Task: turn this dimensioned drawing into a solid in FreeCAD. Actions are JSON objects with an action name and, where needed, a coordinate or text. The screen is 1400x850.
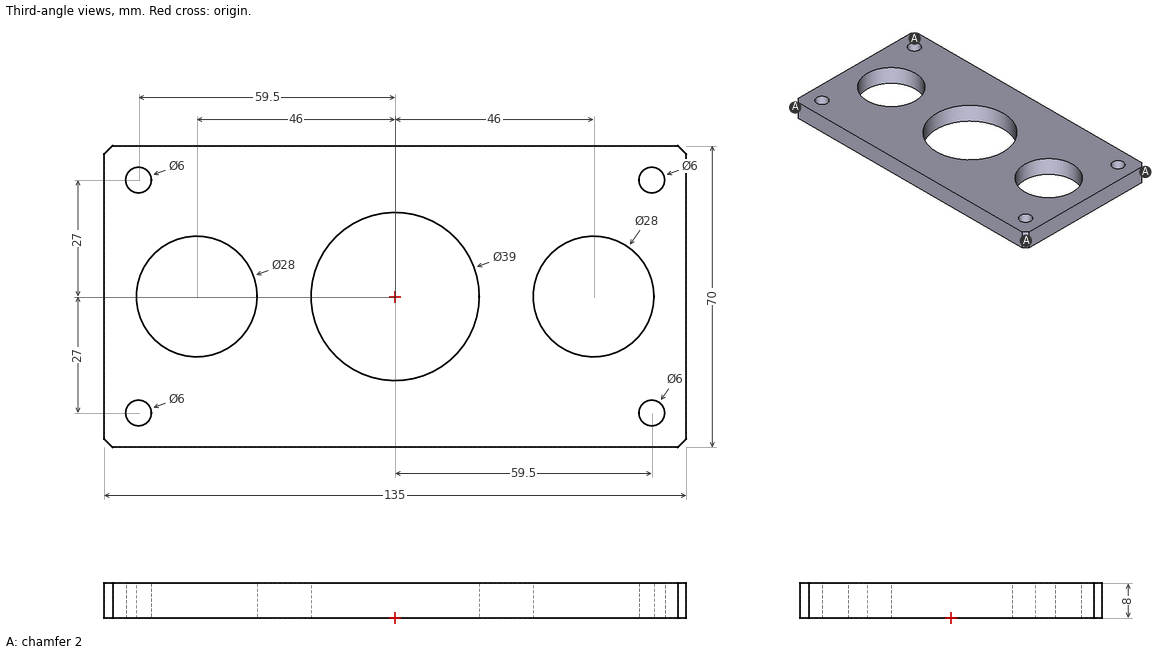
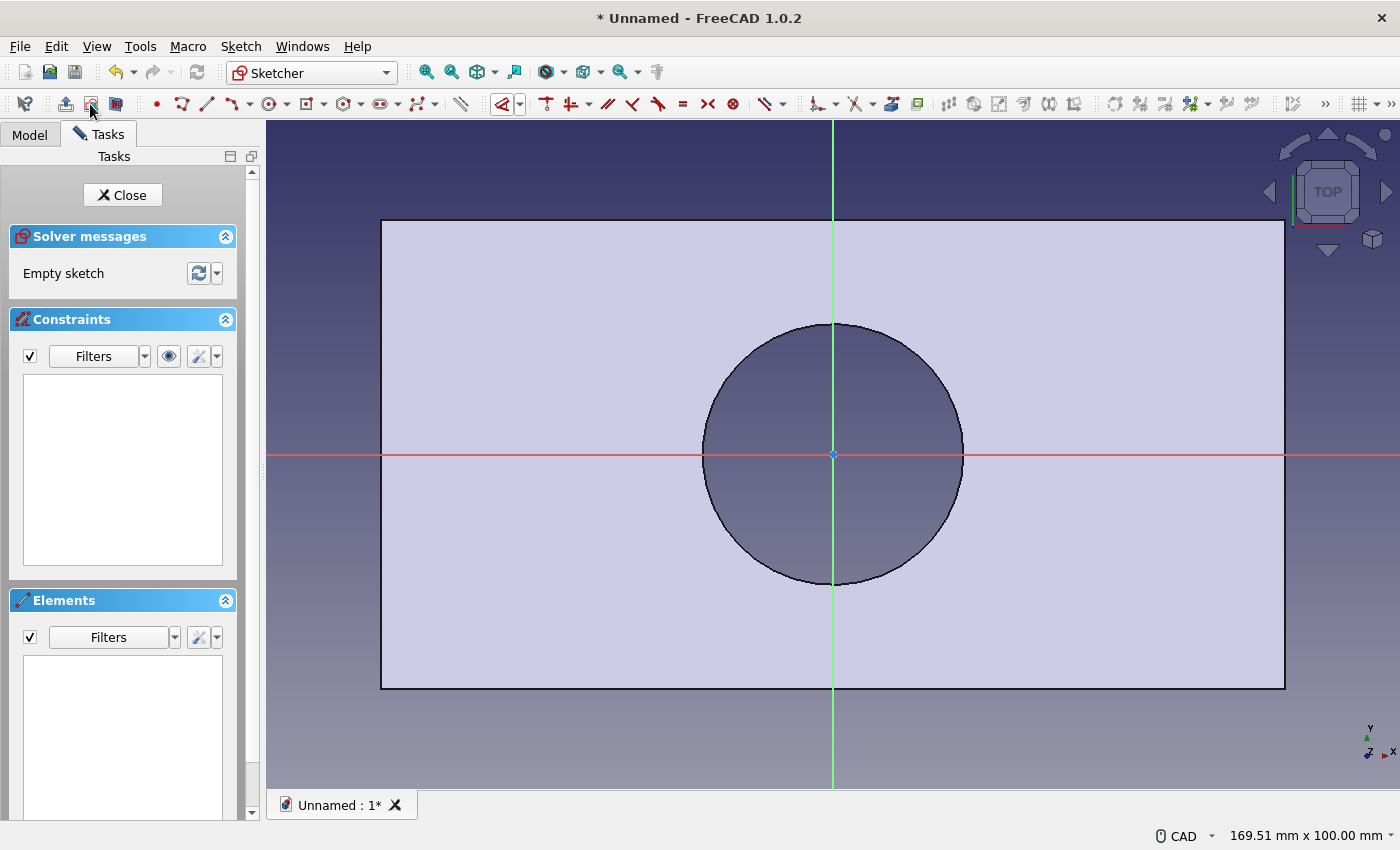
{"action": "scroll", "coordinate": [764, 454], "scroll_direction": "down", "scroll_amount": 5}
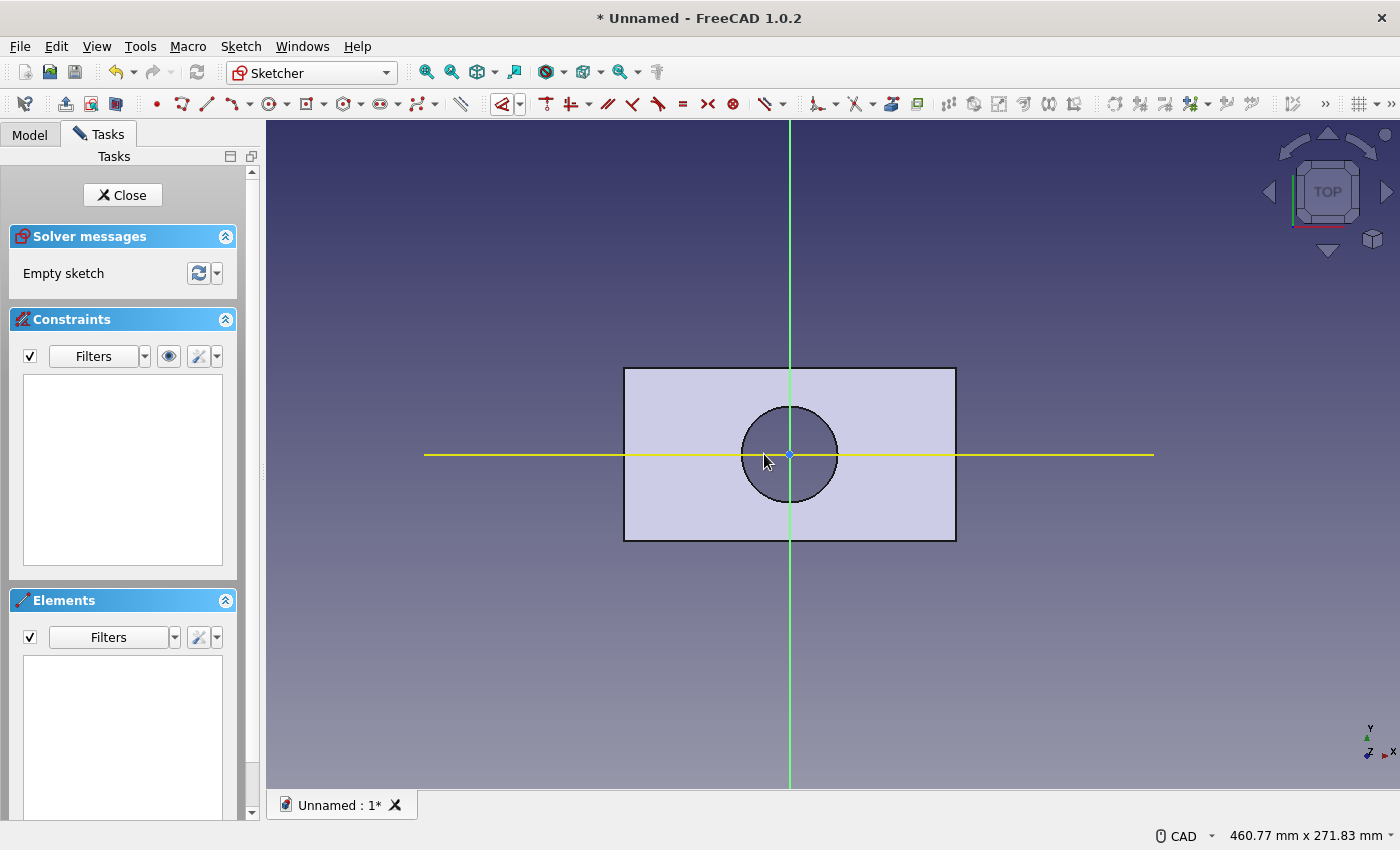
{"action": "scroll", "coordinate": [889, 454], "scroll_direction": "up", "scroll_amount": 8}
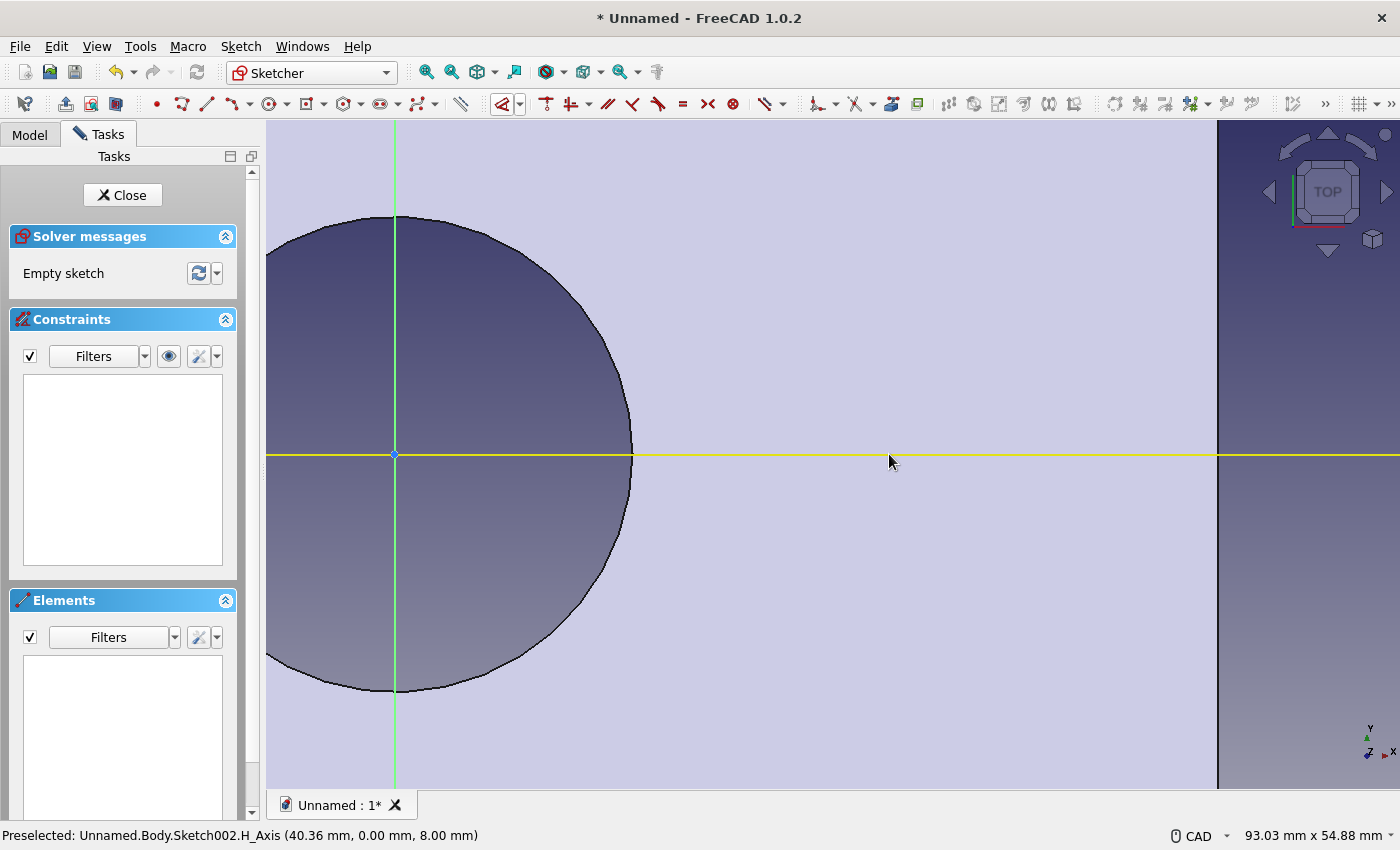
{"action": "left_click", "coordinate": [268, 104]}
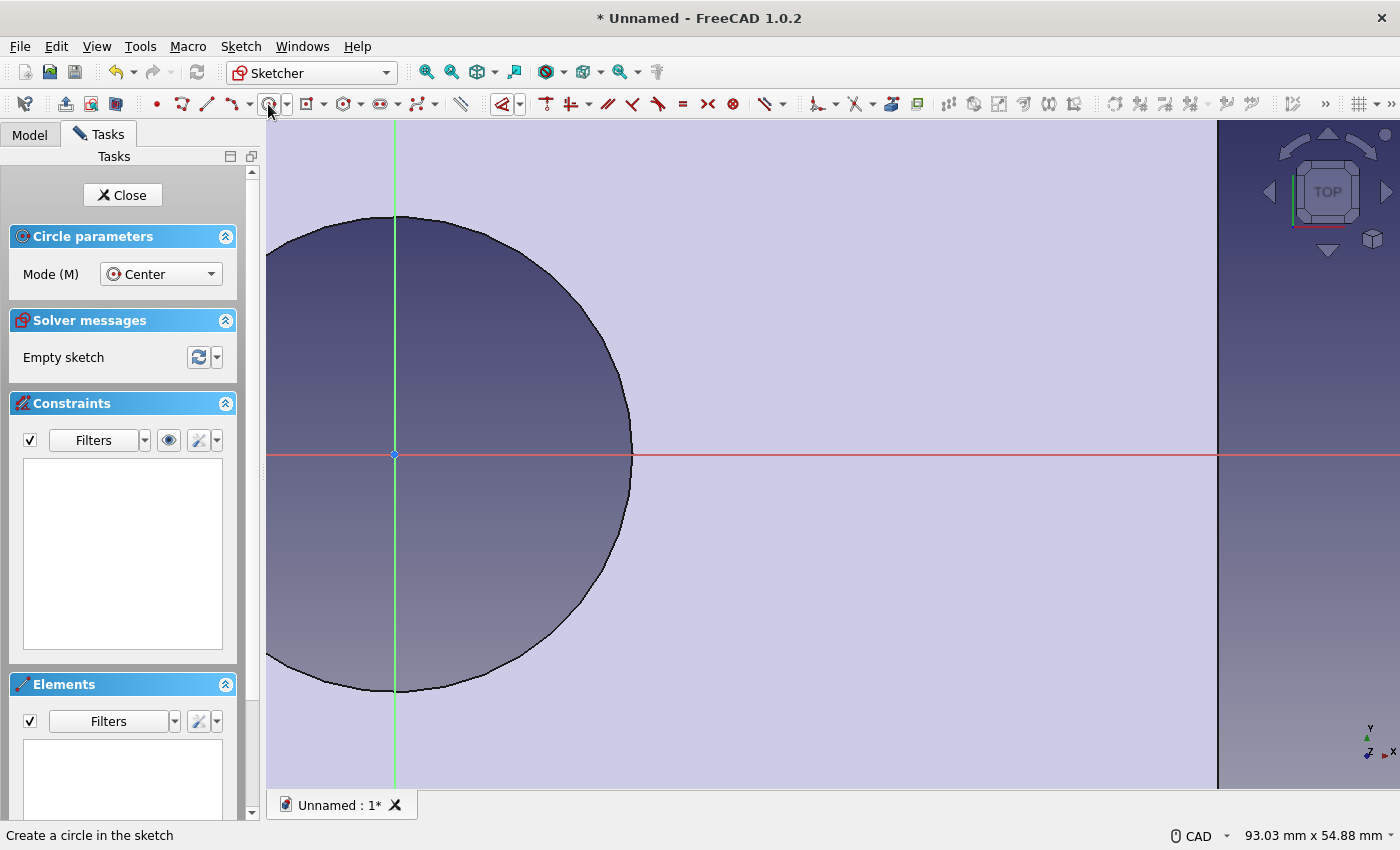
{"action": "left_click", "coordinate": [956, 454]}
{"action": "left_click", "coordinate": [1076, 334]}
{"action": "key", "text": "Escape"}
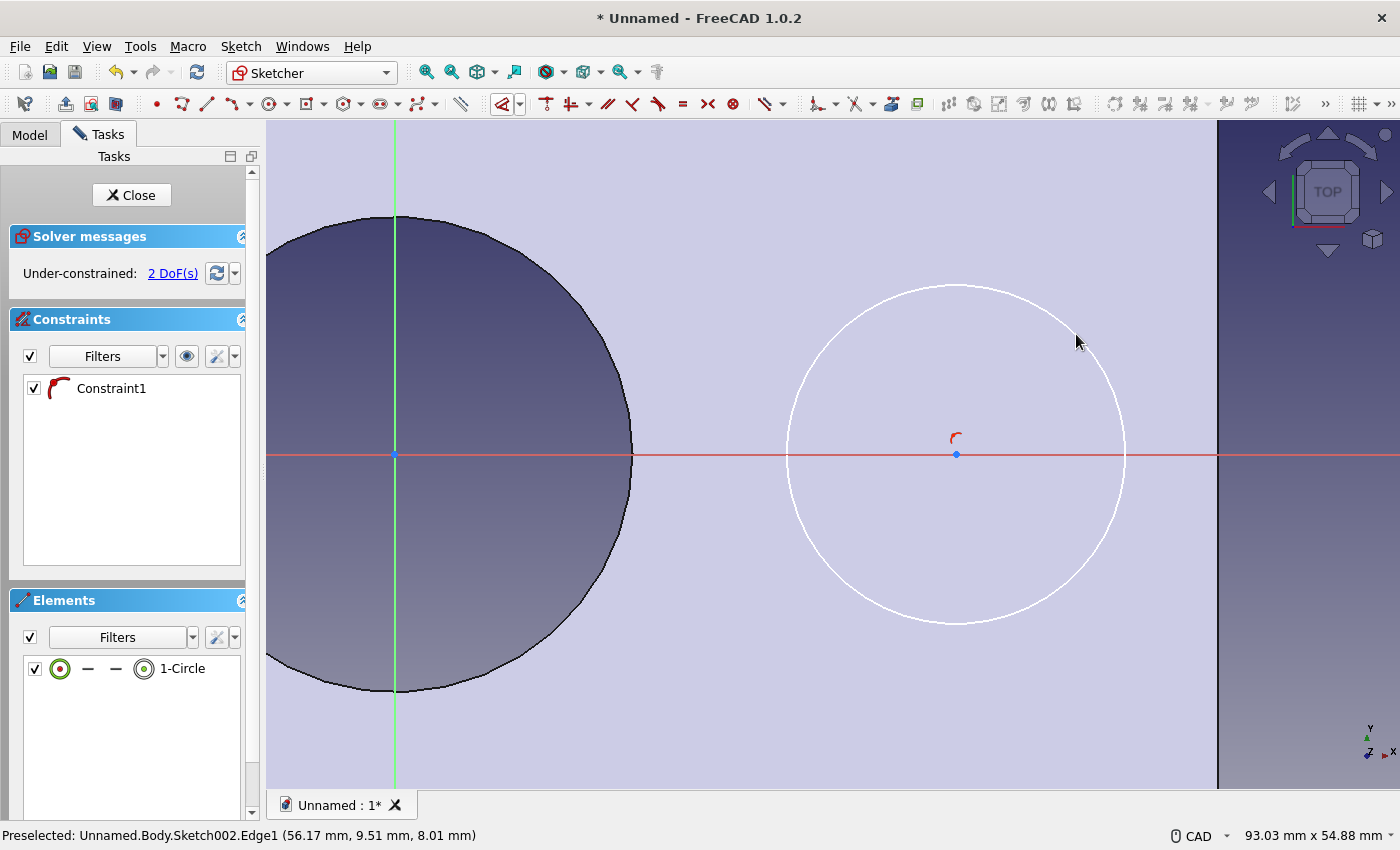
{"action": "left_click", "coordinate": [1075, 334]}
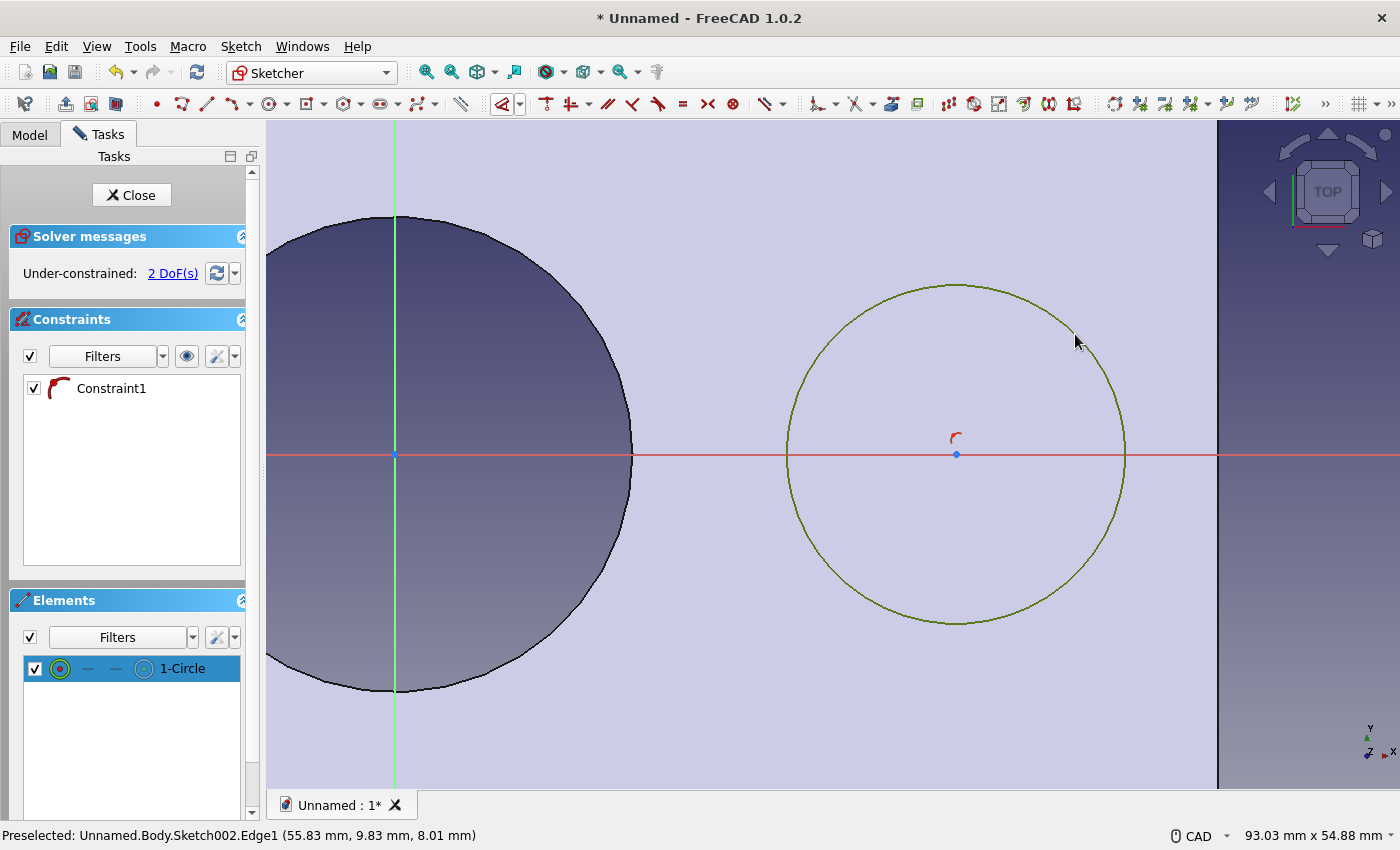
{"action": "key", "text": "k o"}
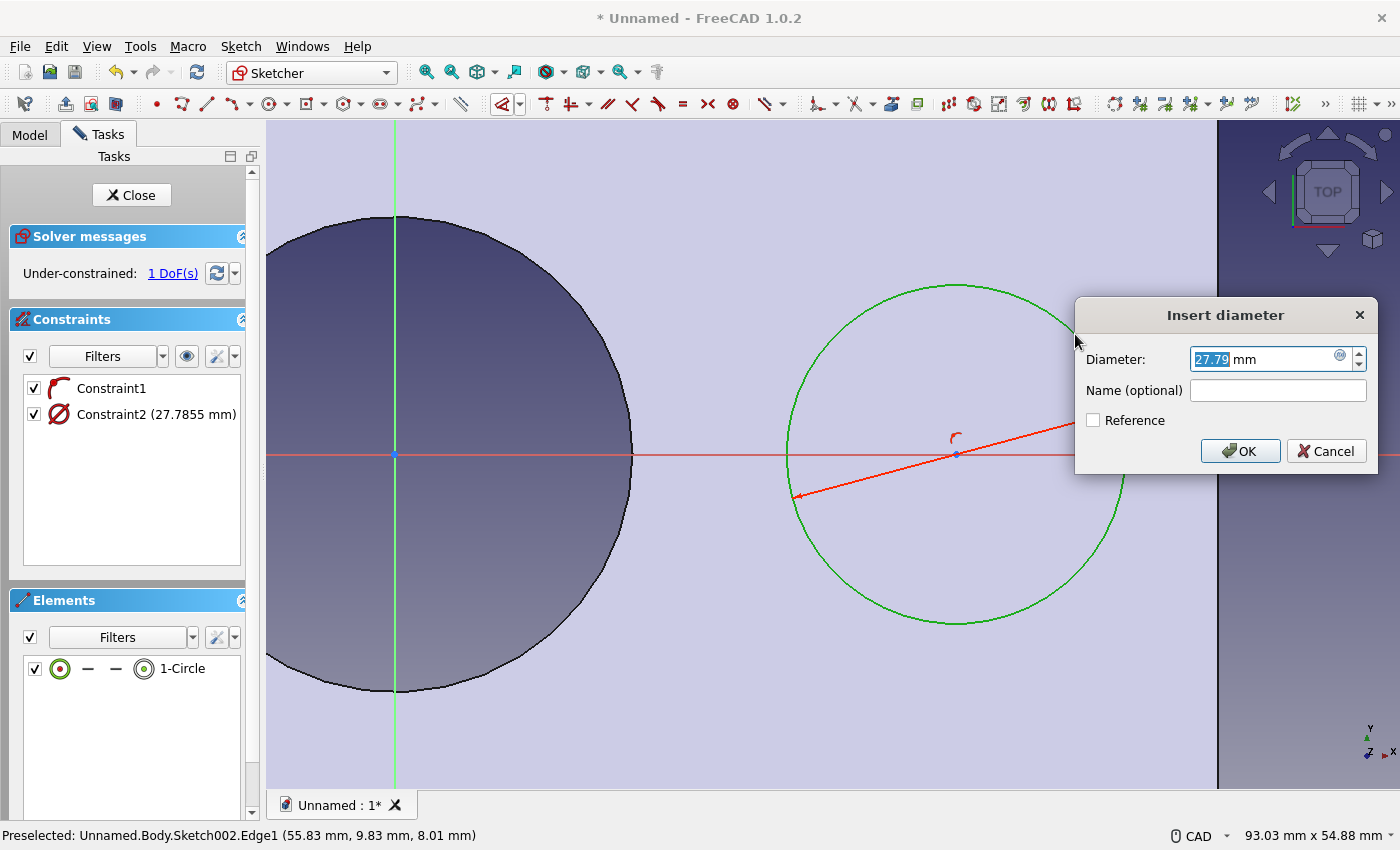
{"action": "type", "text": "28"}
{"action": "key", "text": "Return"}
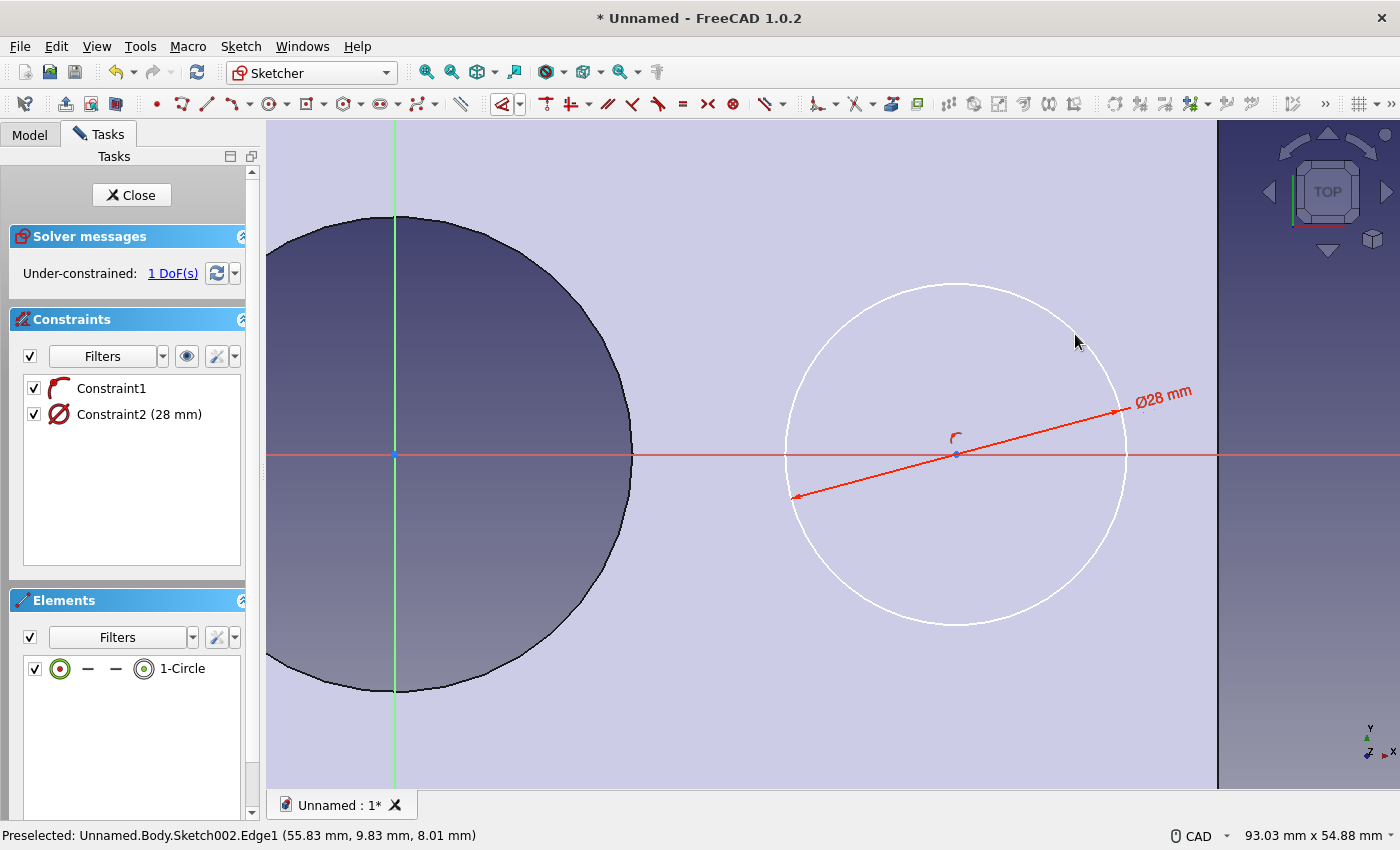
{"action": "left_click", "coordinate": [956, 454]}